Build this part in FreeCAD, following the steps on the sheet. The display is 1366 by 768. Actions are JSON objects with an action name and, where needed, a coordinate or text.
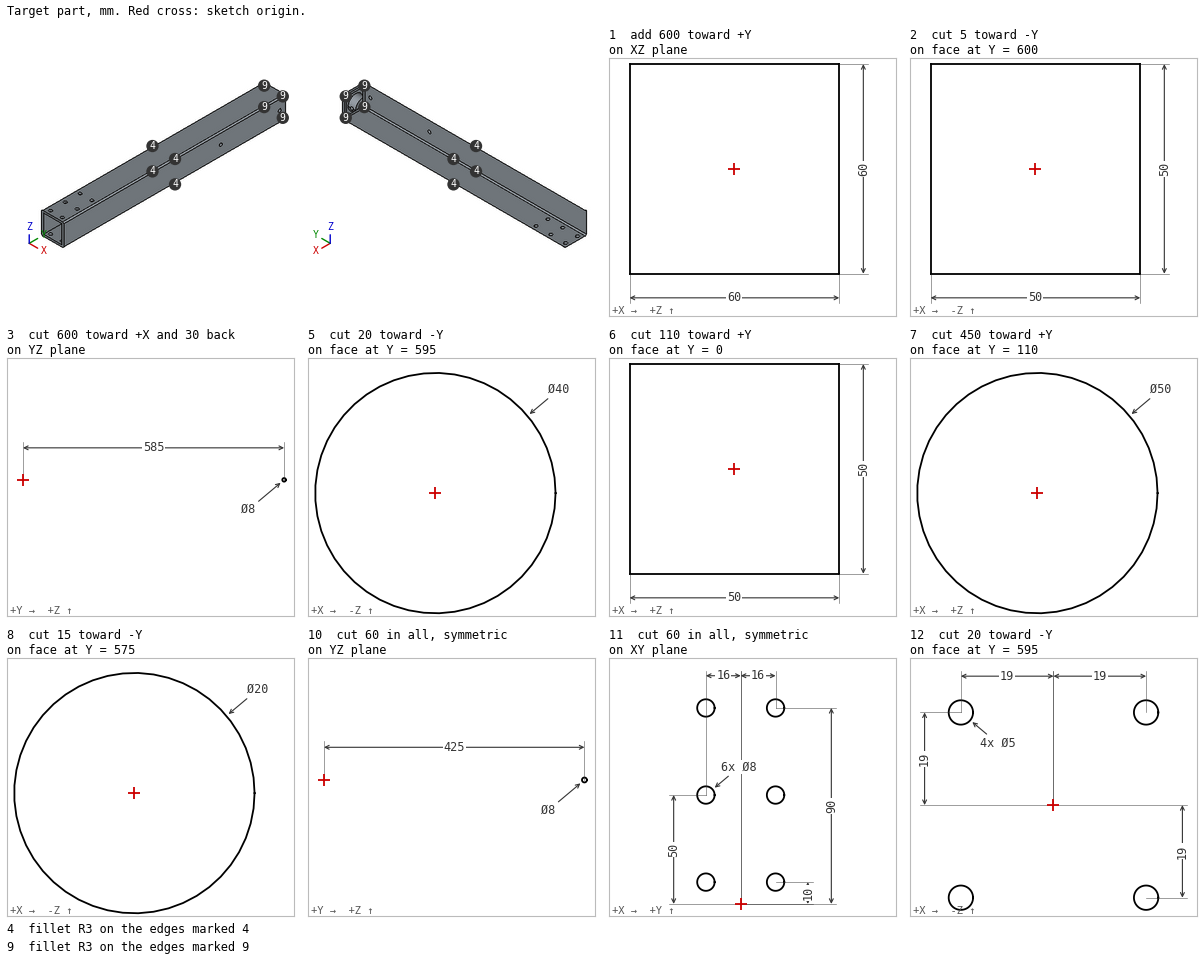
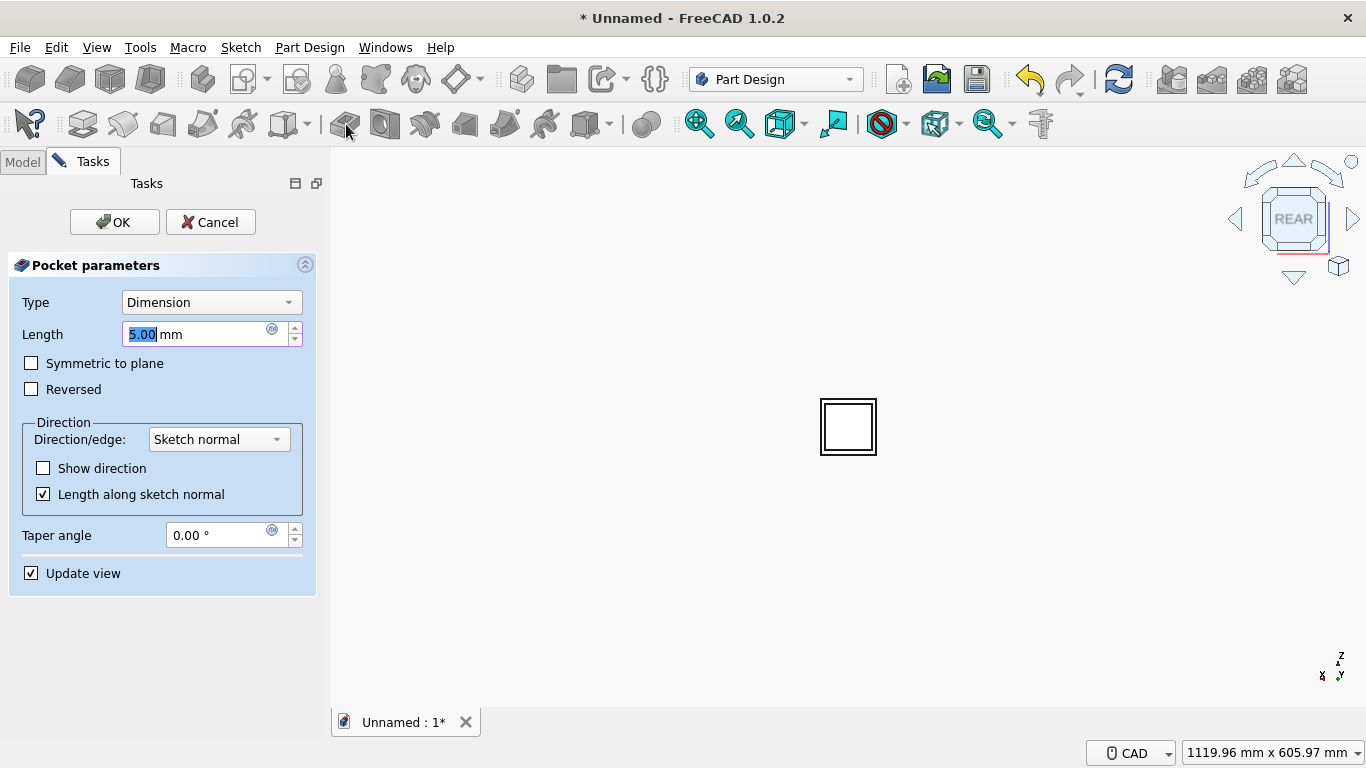
{"action": "left_click", "coordinate": [212, 302]}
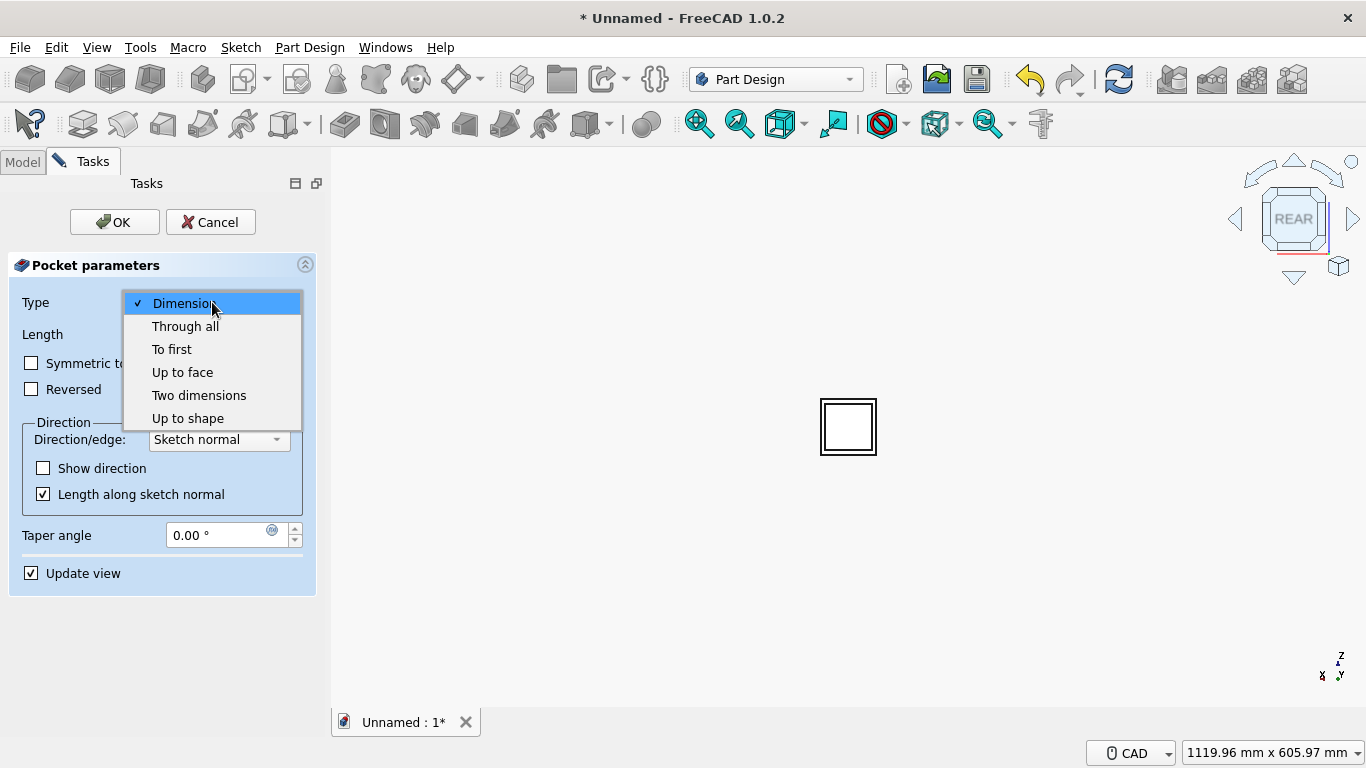
{"action": "left_click", "coordinate": [212, 396]}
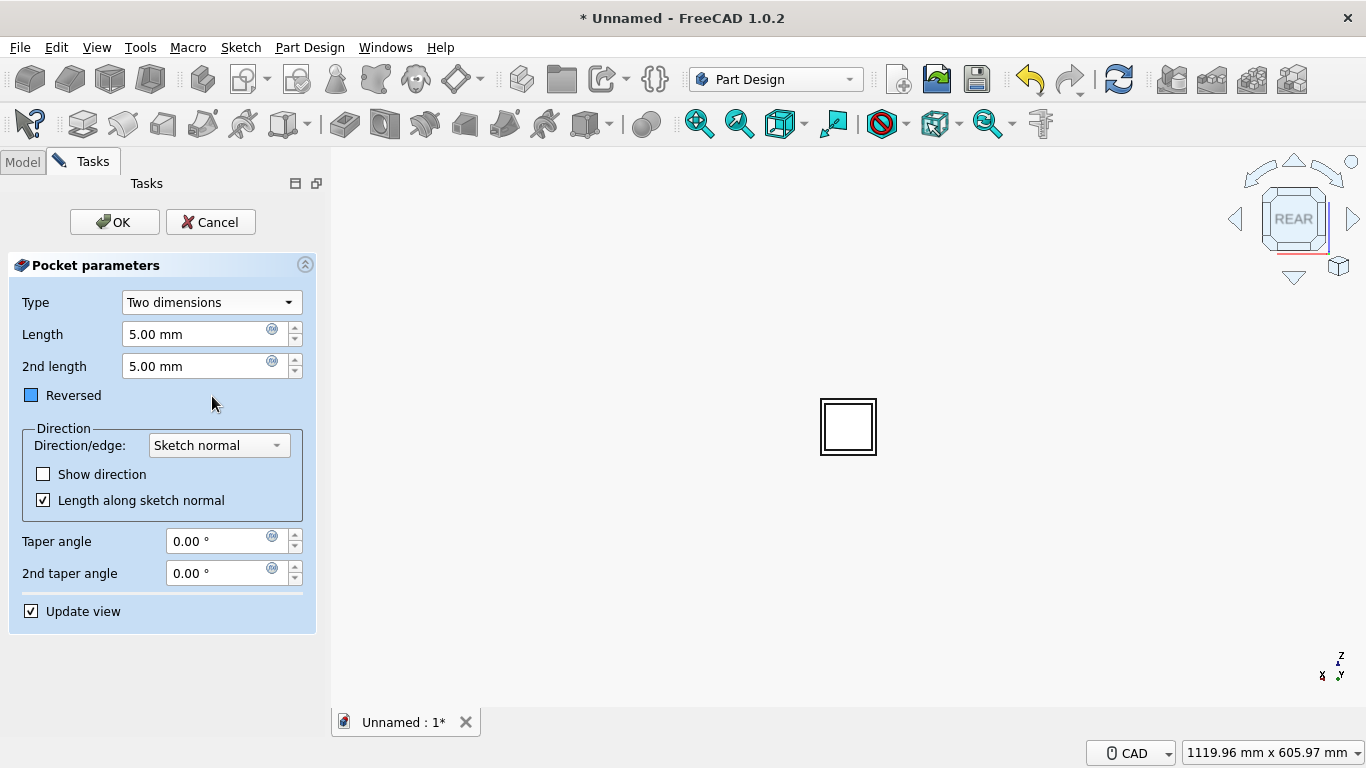
{"action": "triple_click", "coordinate": [204, 334]}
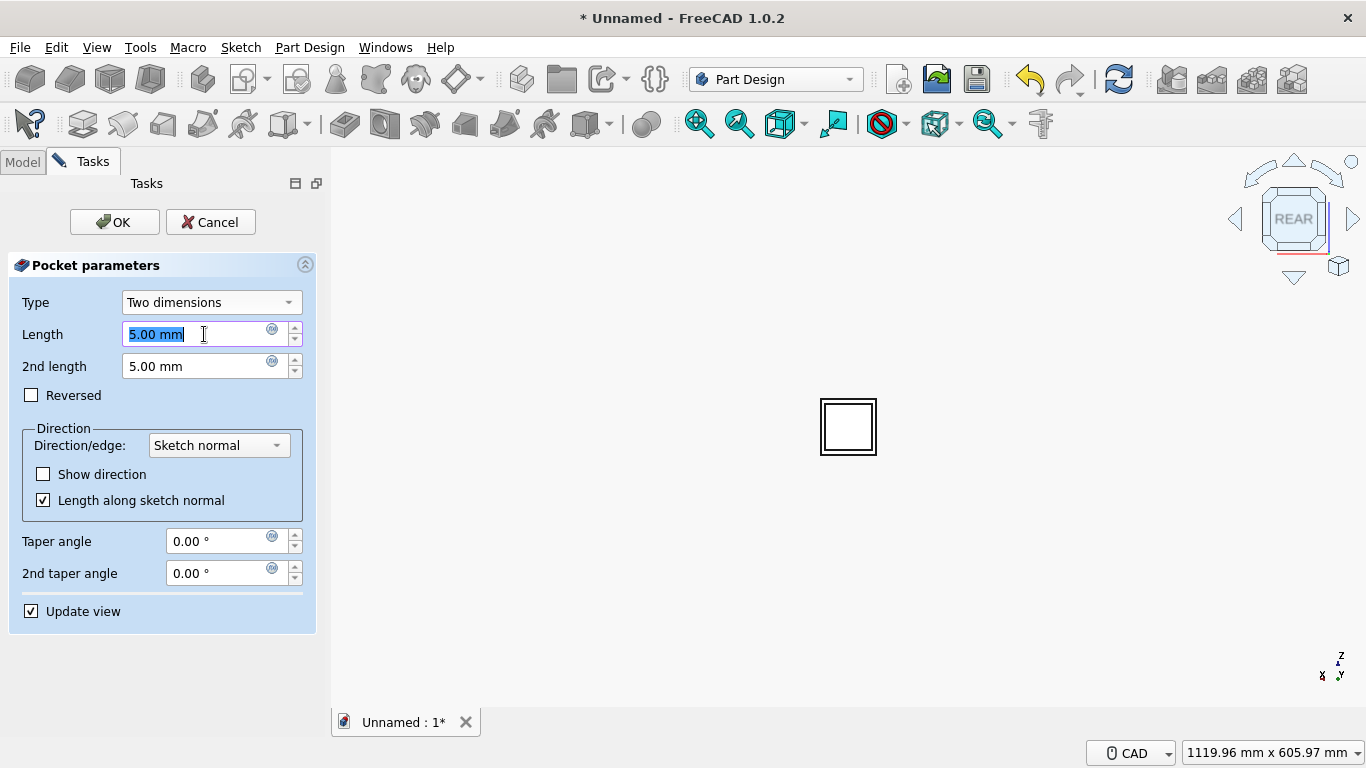
{"action": "type", "text": "600"}
{"action": "key", "text": "Tab"}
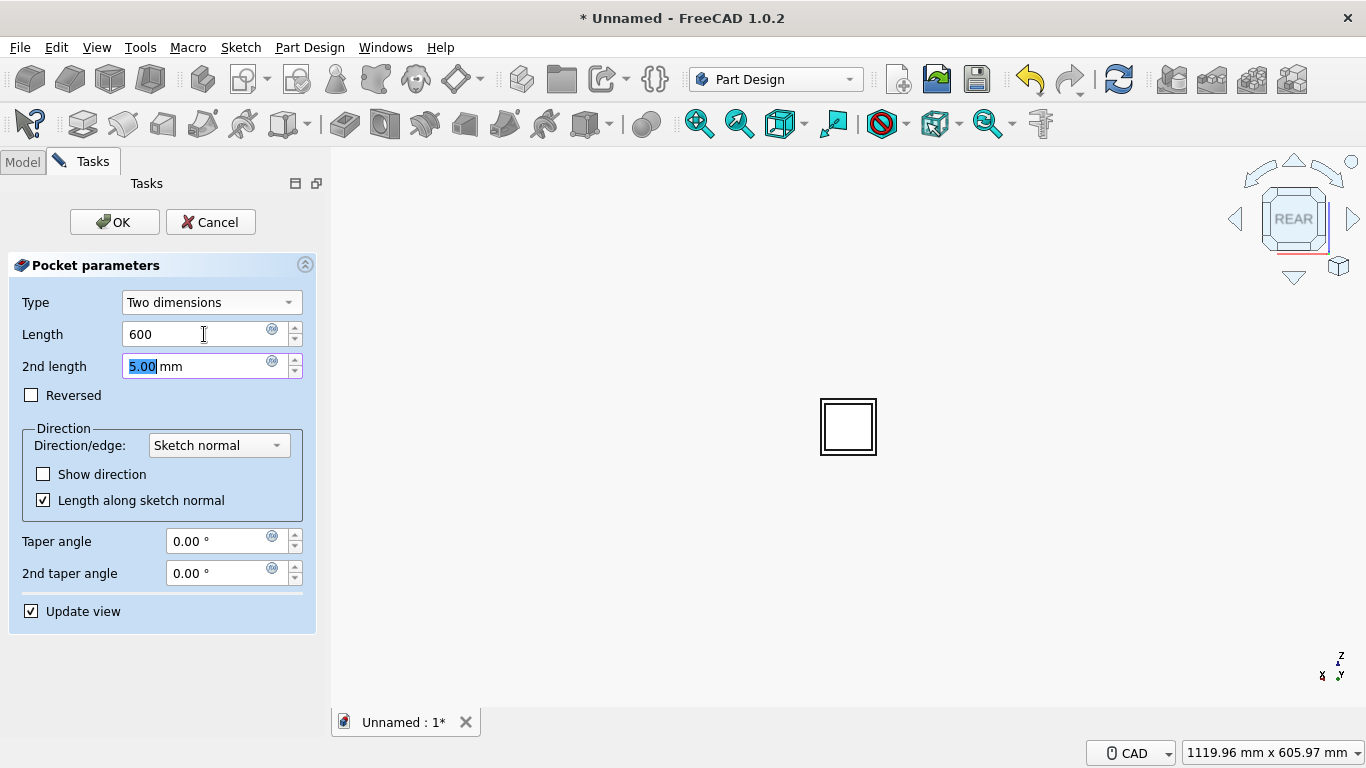
{"action": "type", "text": "30"}
{"action": "key", "text": "Tab"}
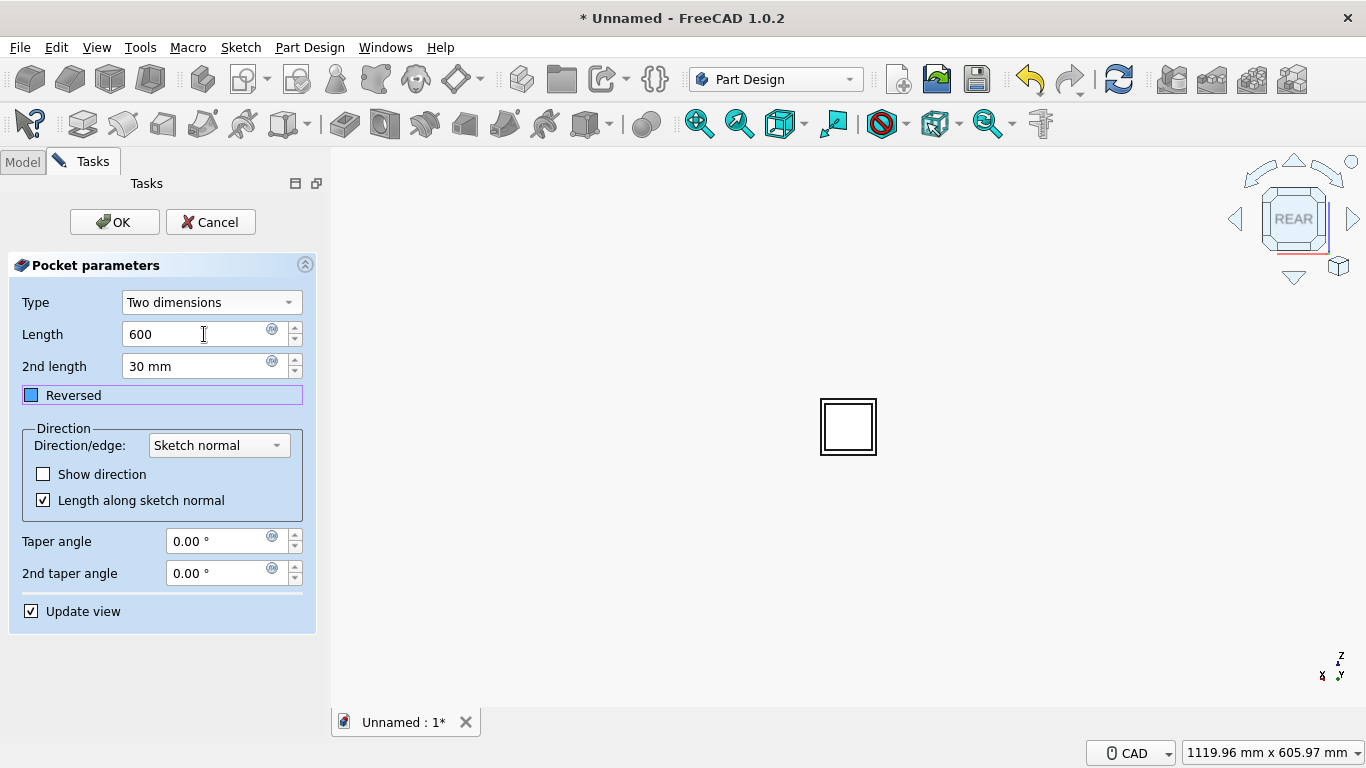
{"action": "left_click", "coordinate": [30, 395]}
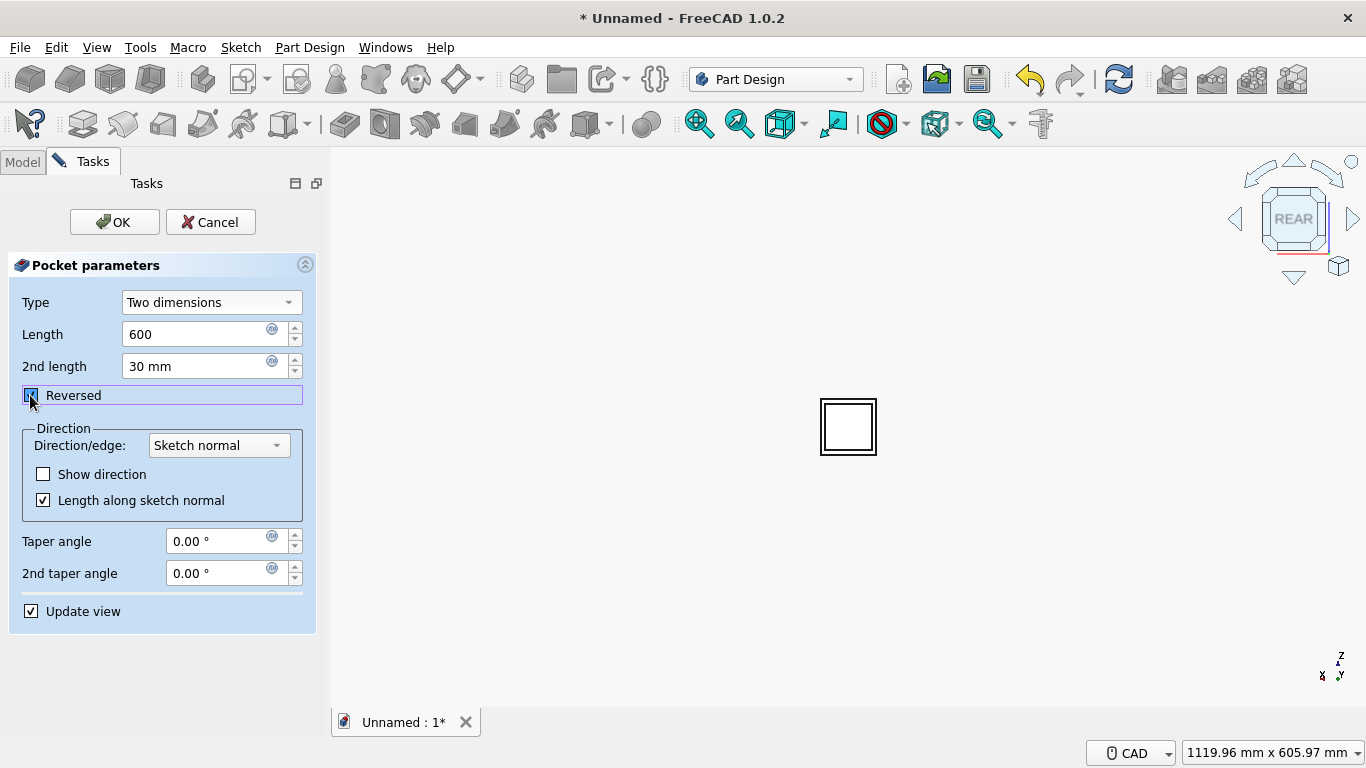
{"action": "left_click", "coordinate": [115, 222]}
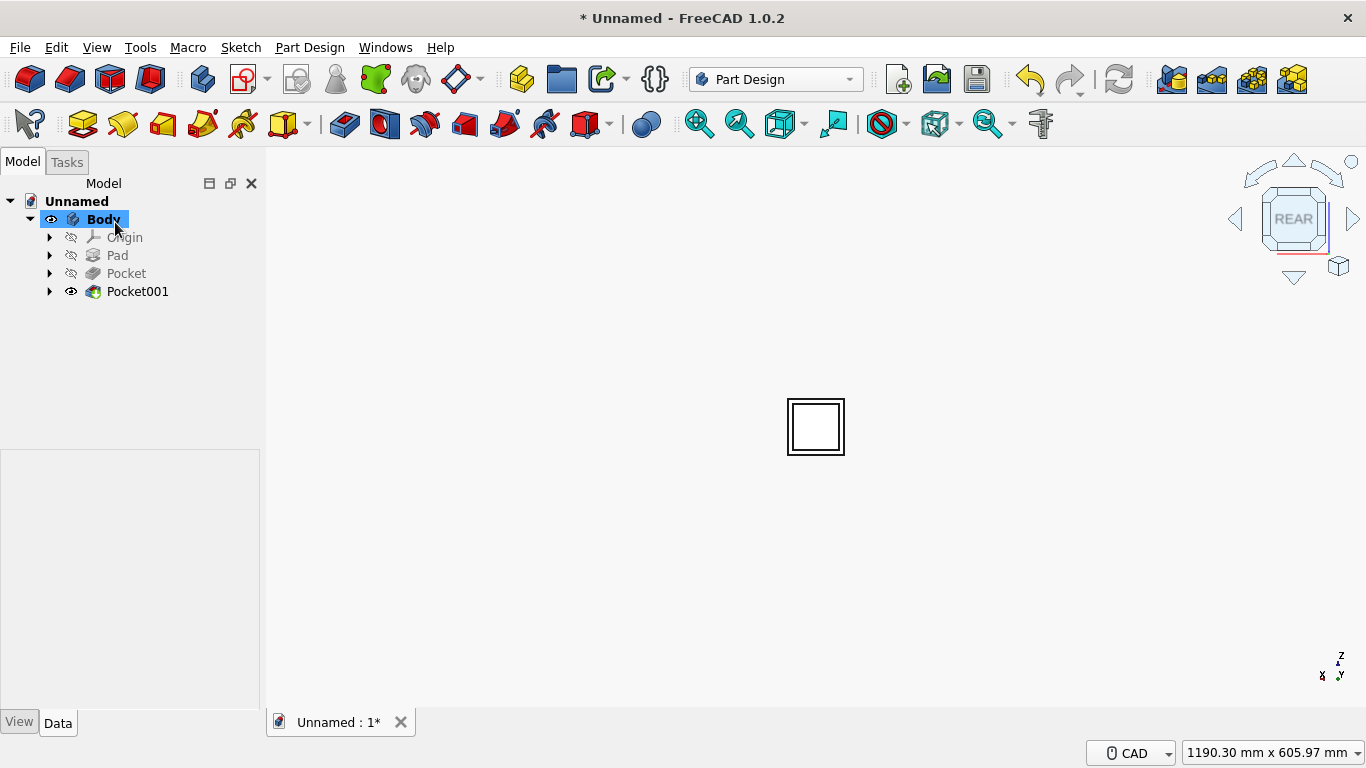
{"action": "left_click", "coordinate": [700, 124]}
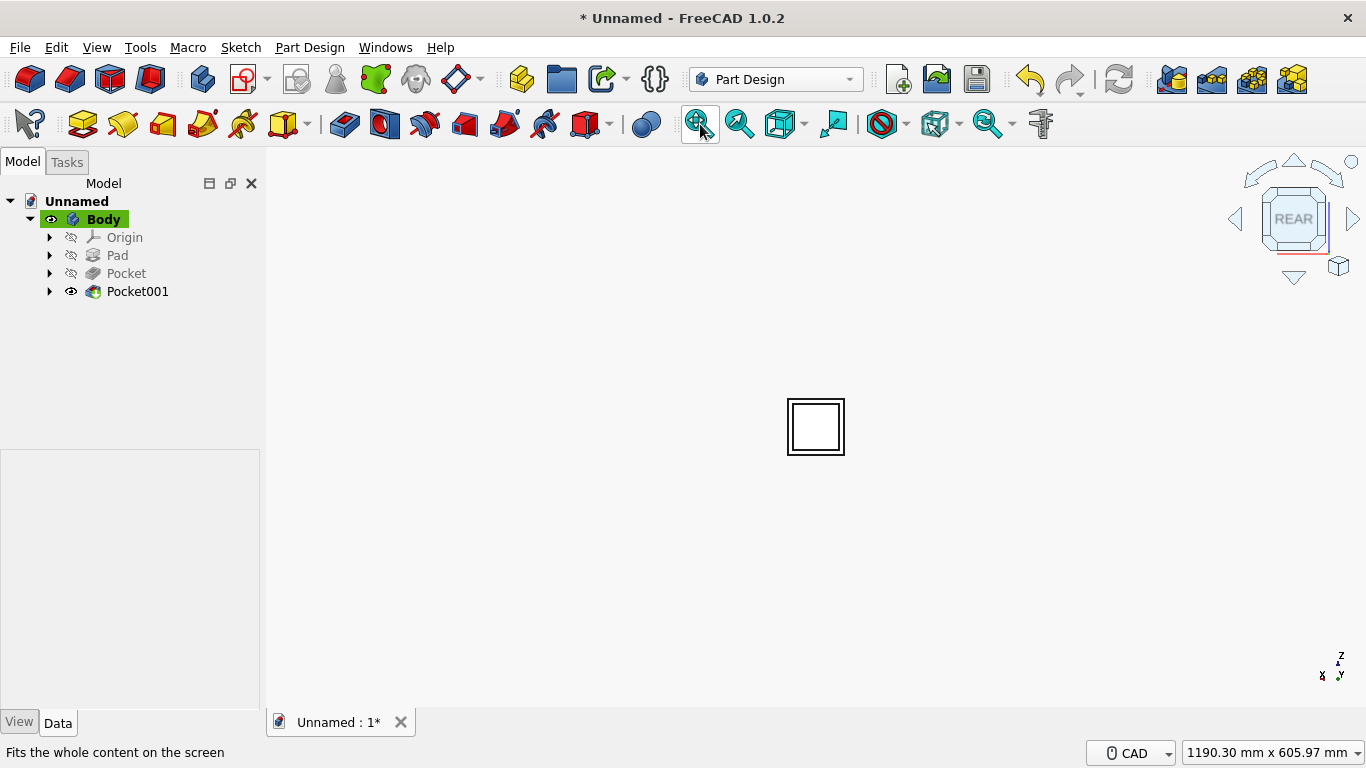
{"action": "key", "text": "0"}